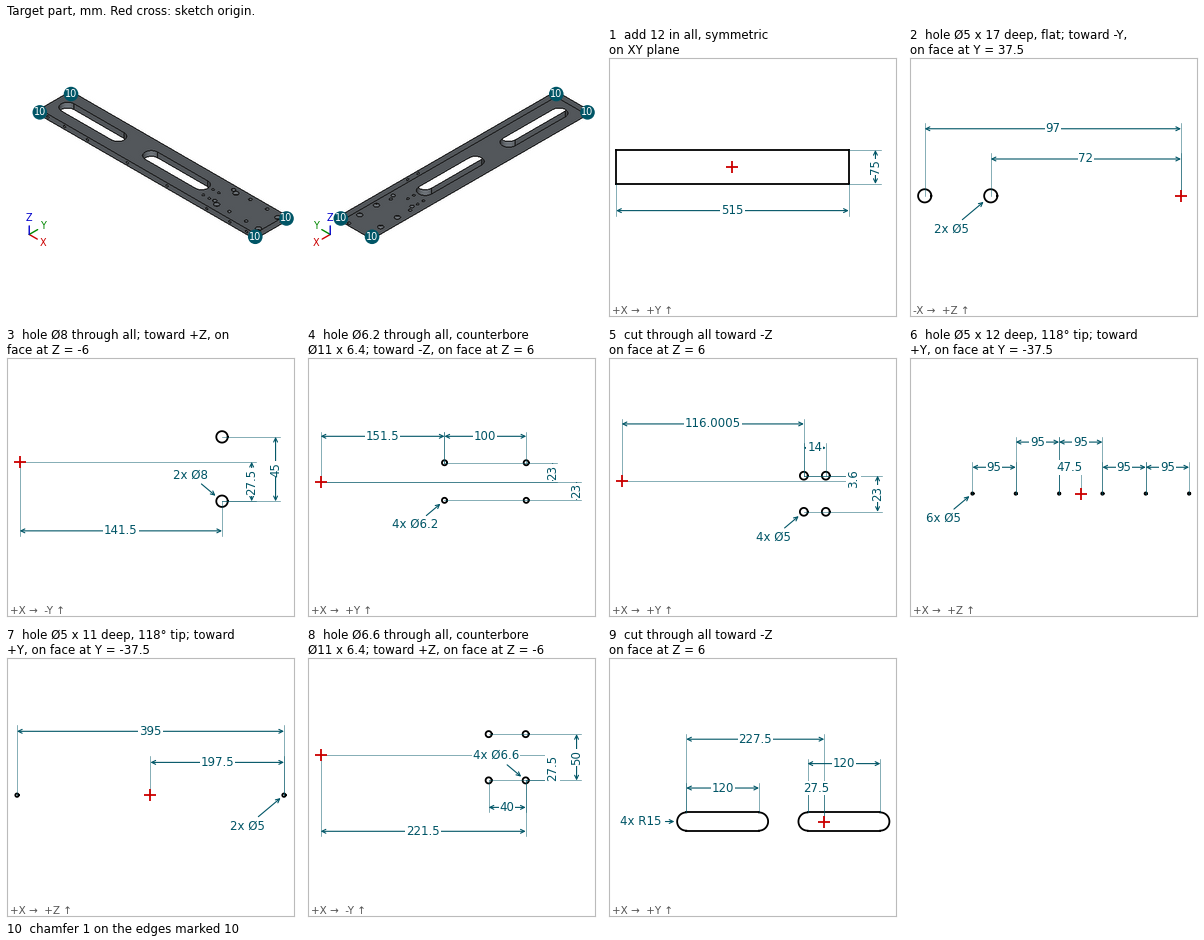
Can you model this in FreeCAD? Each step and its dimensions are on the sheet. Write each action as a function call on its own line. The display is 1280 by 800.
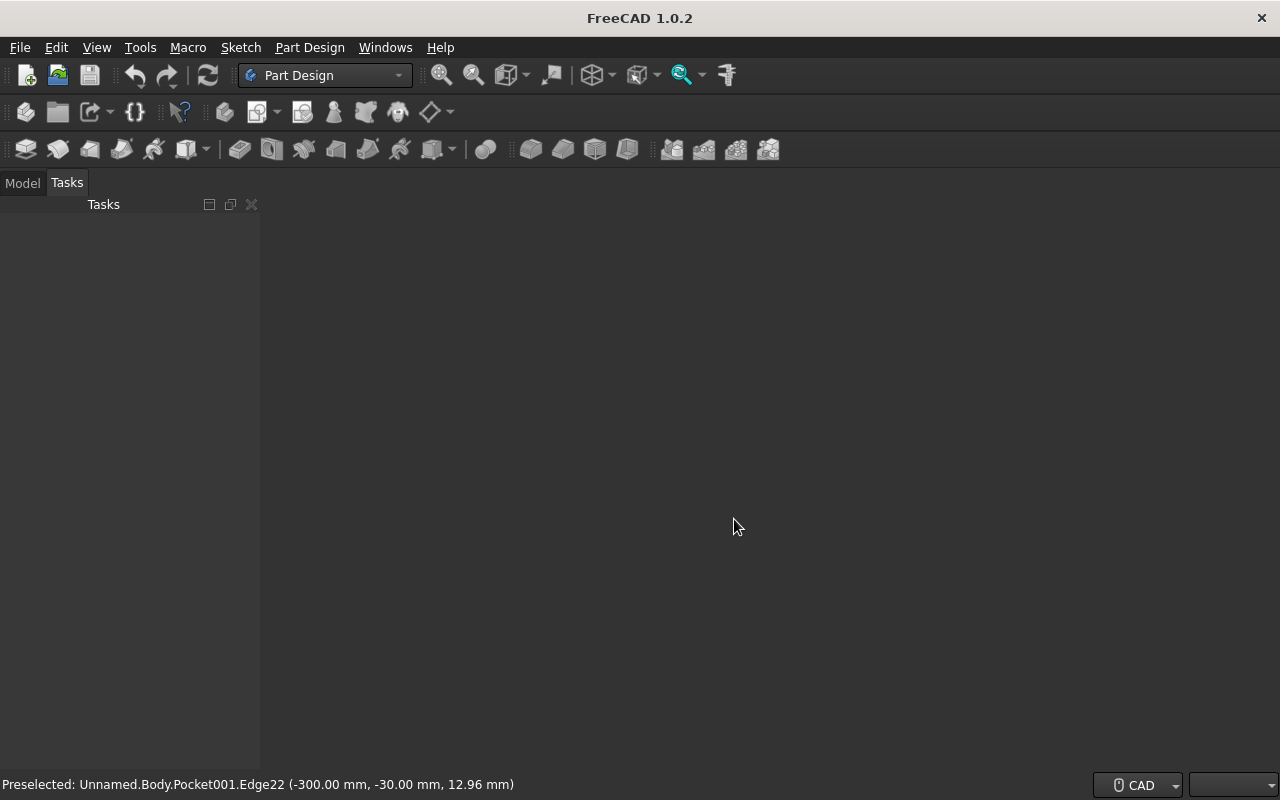
key(ctrl+n)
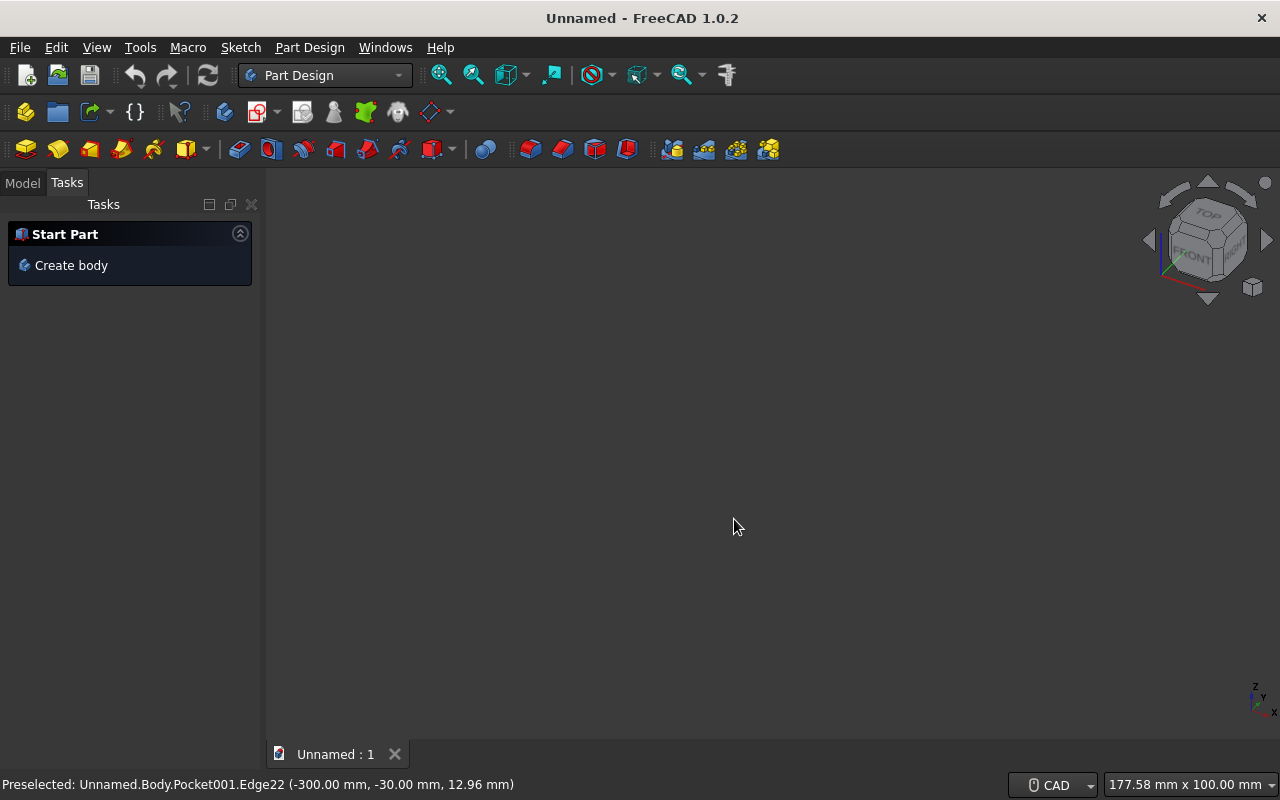
click(258, 112)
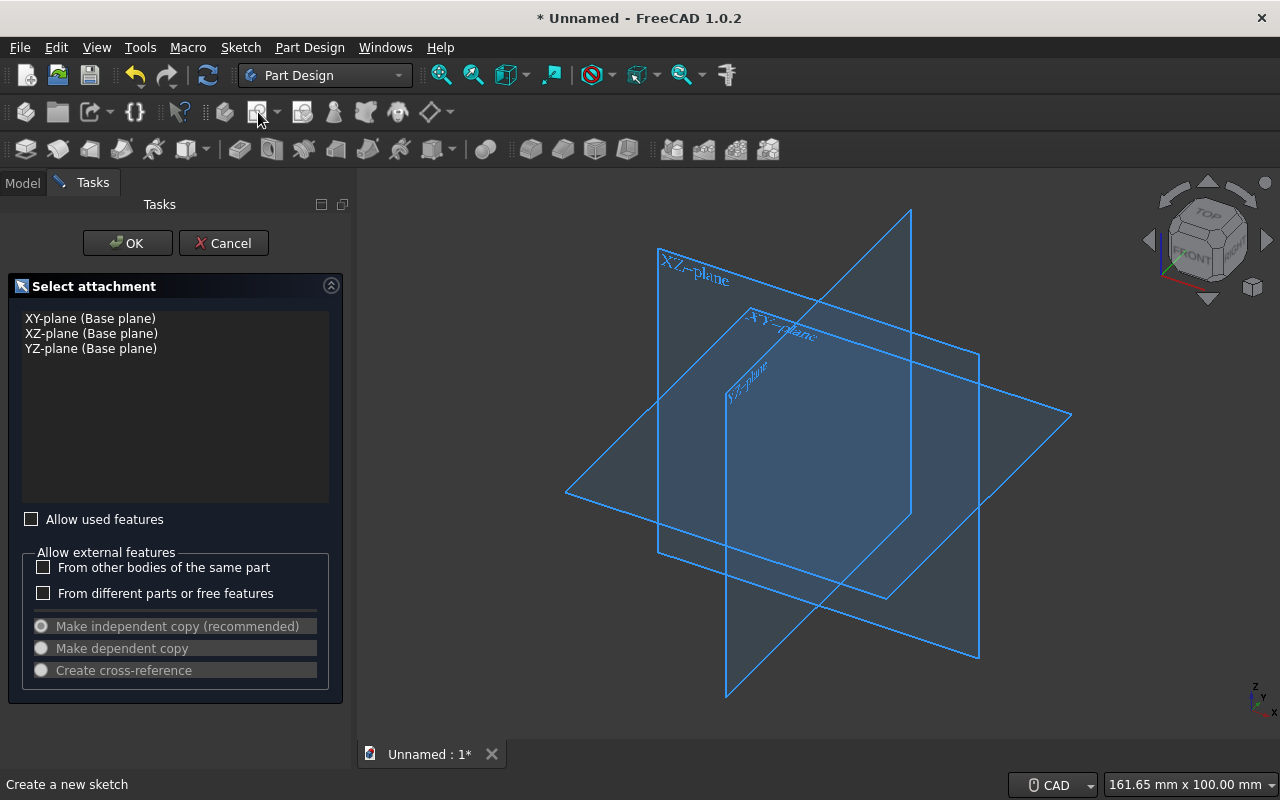
click(82, 318)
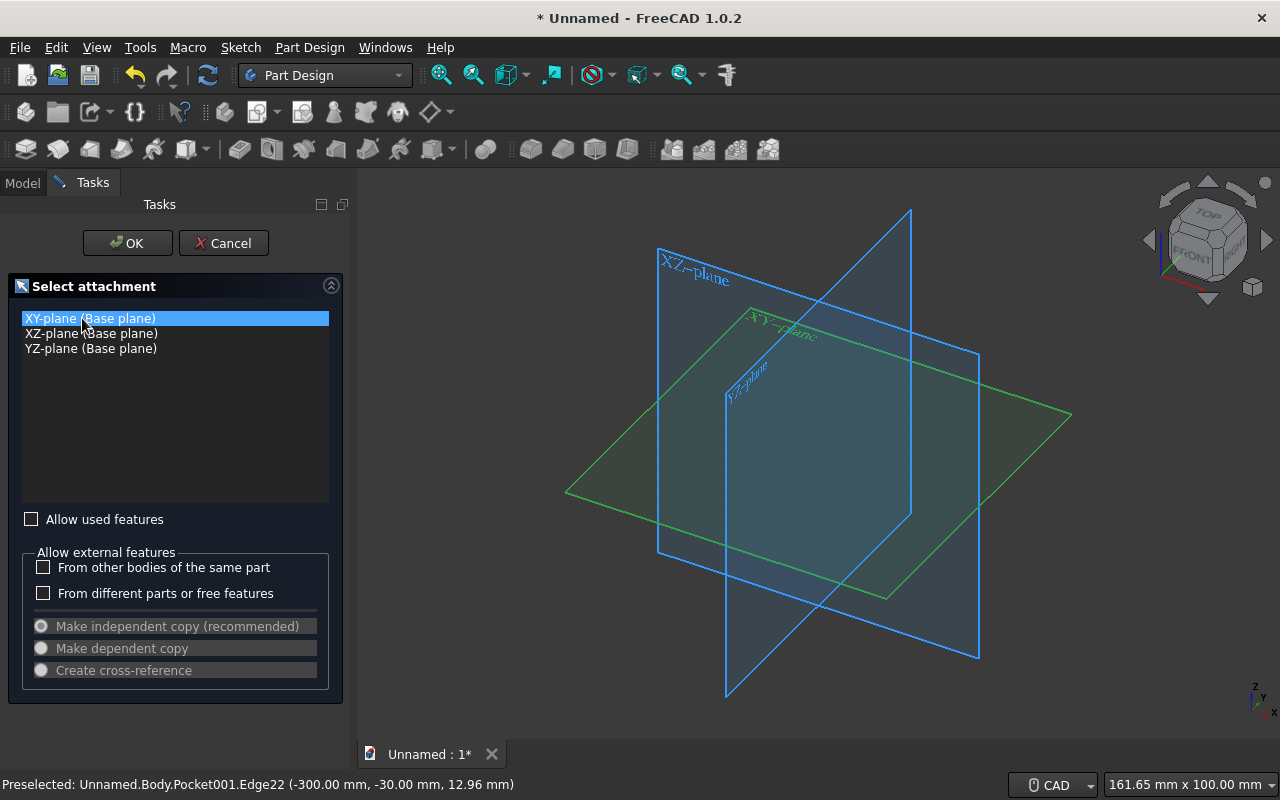
click(128, 243)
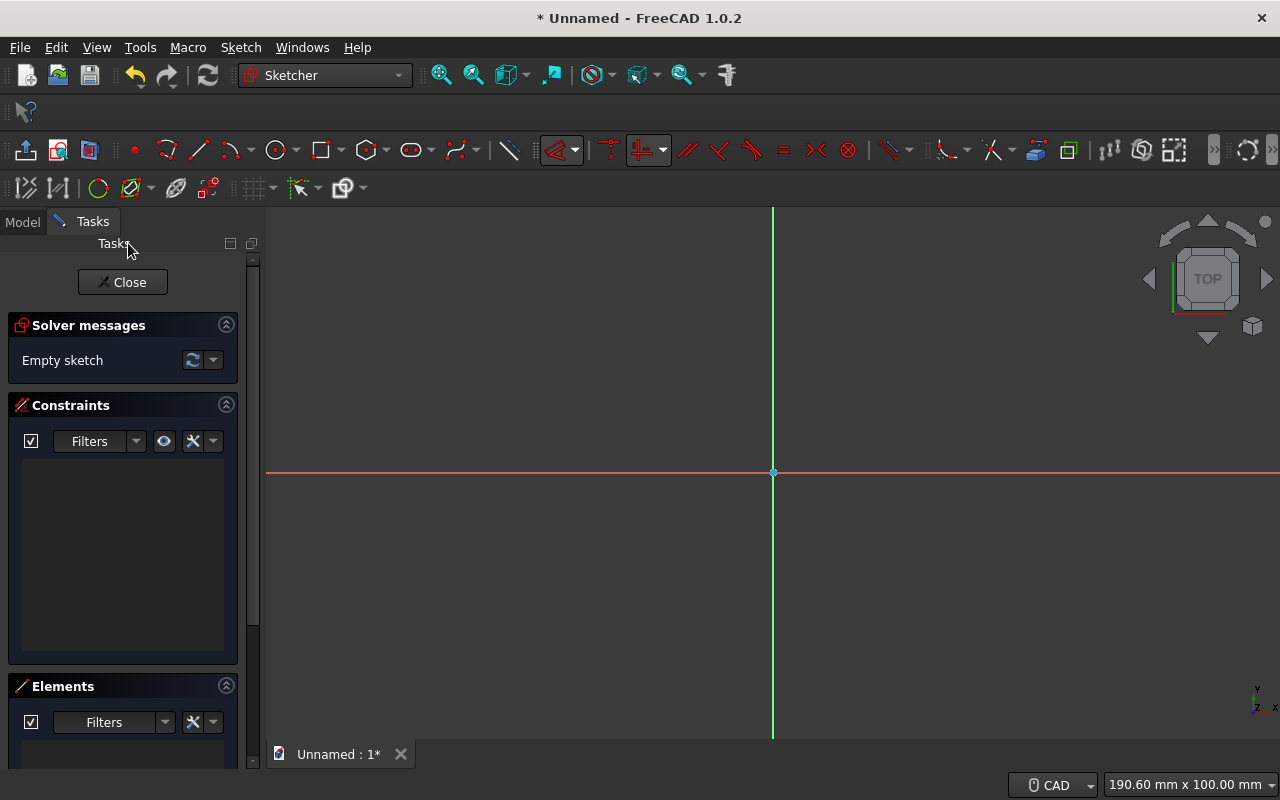
scroll(687, 473, down, 8)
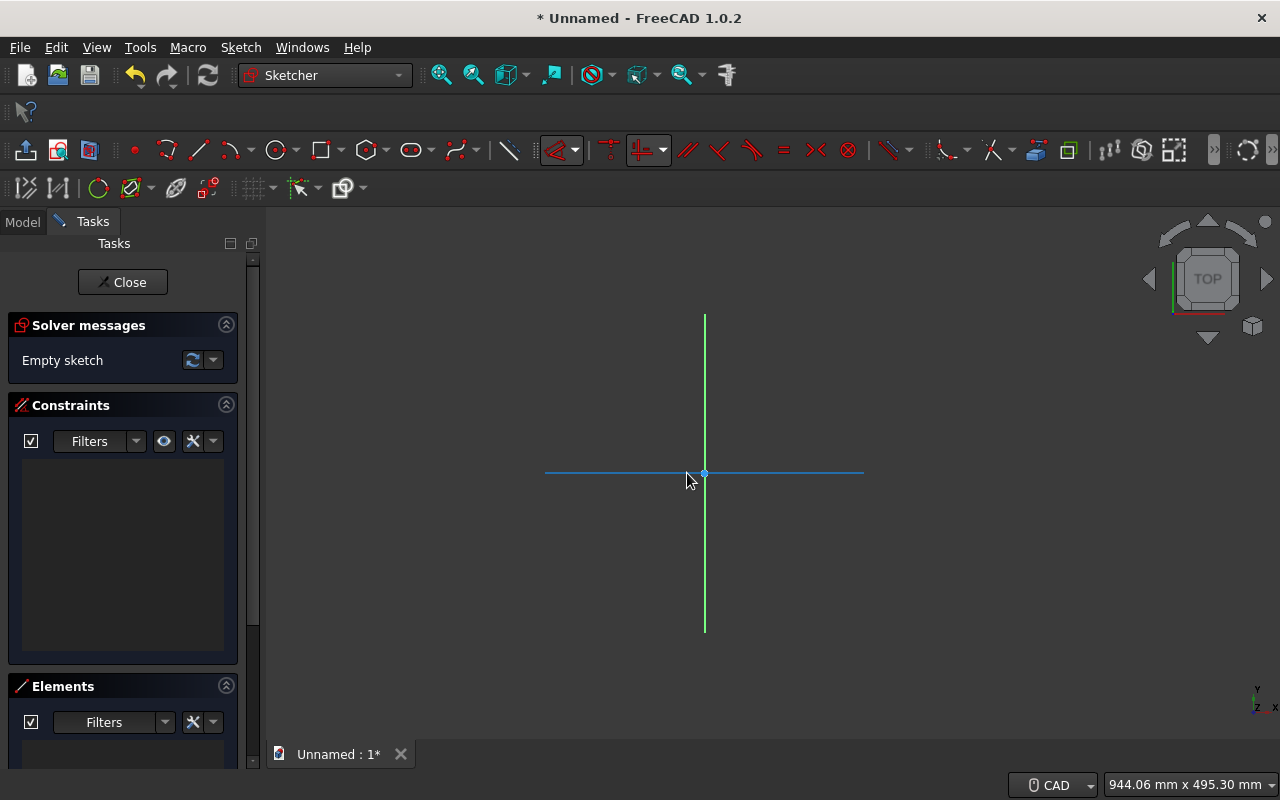
key(g)
key(v)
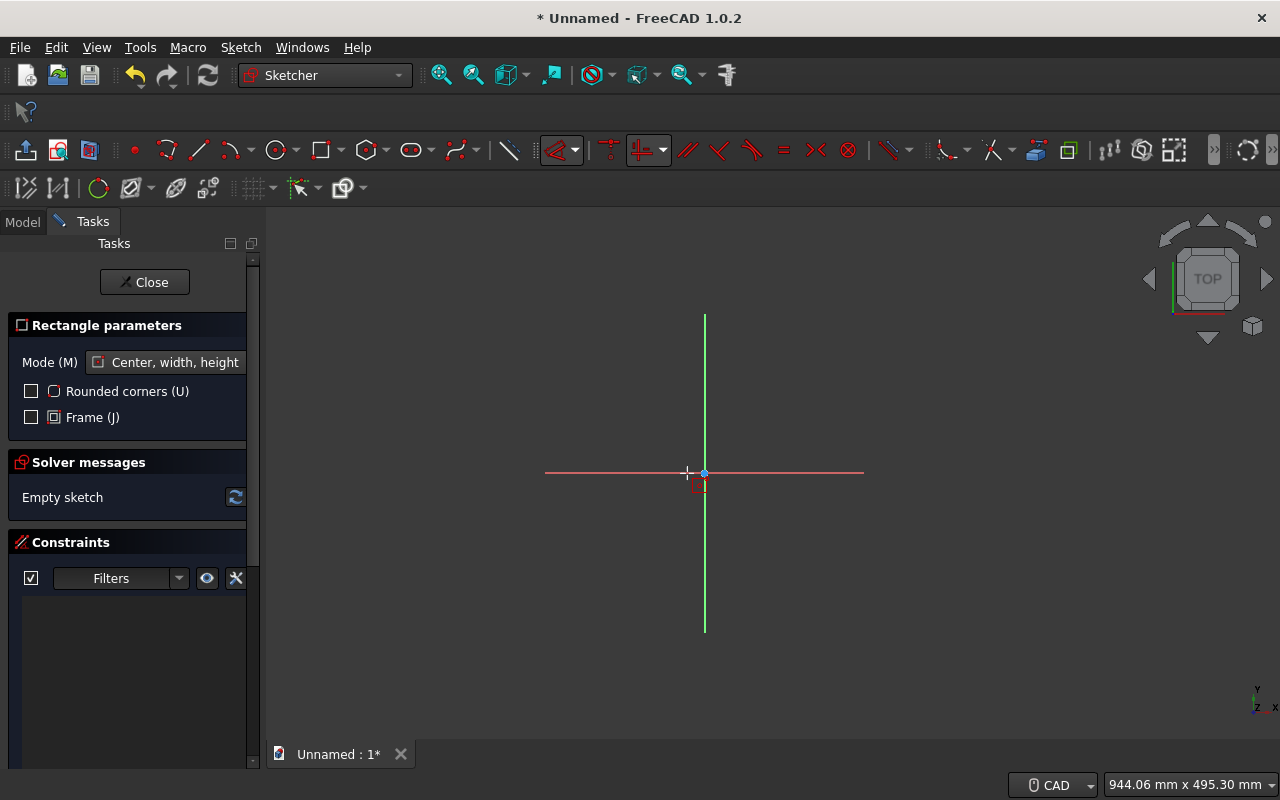
click(705, 473)
click(981, 433)
key(Escape)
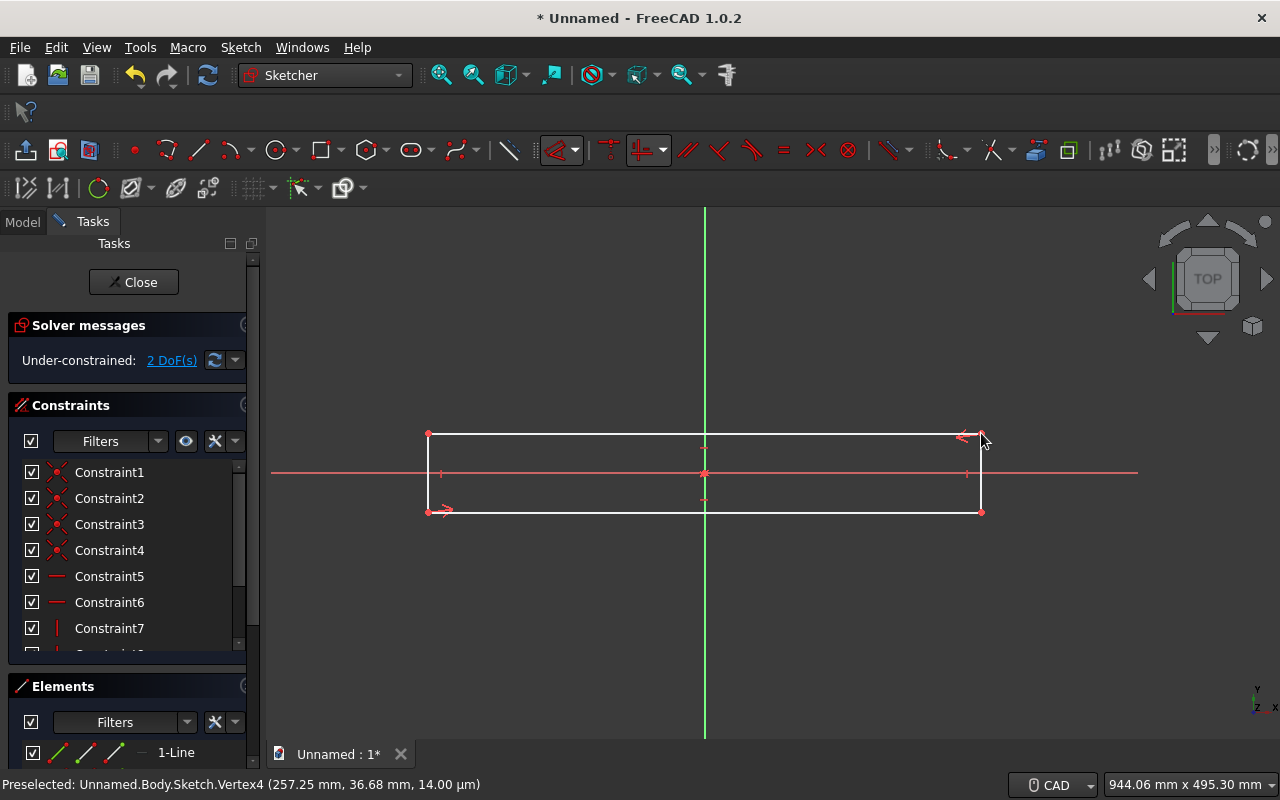
key(d)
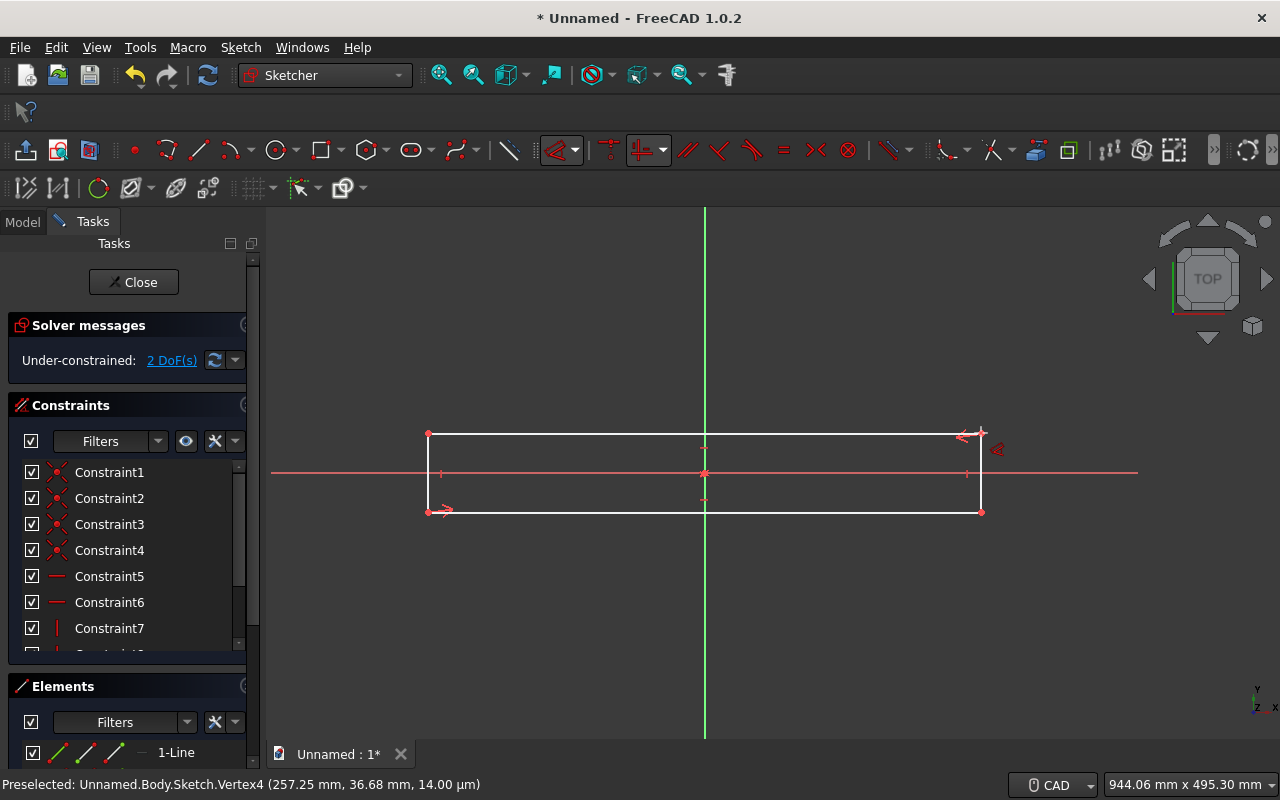
click(981, 489)
click(1015, 455)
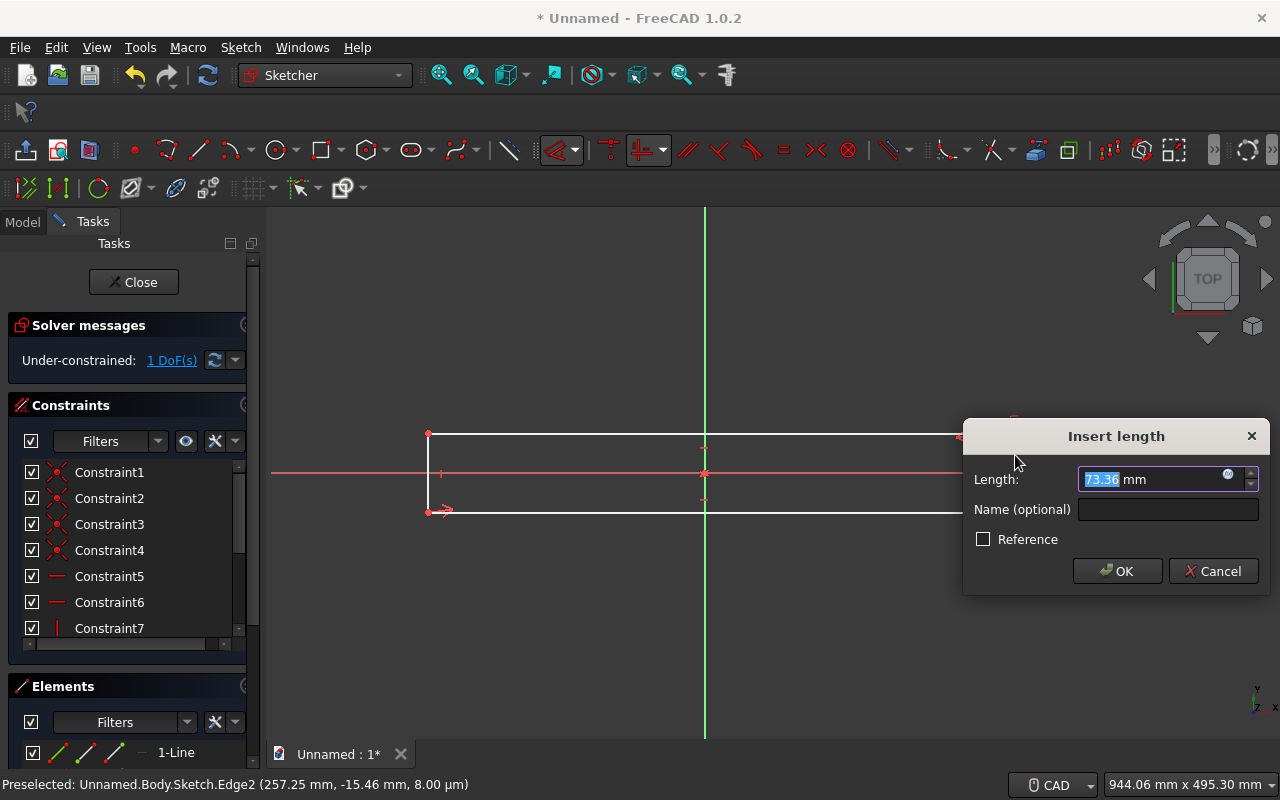
text(75)
key(Return)